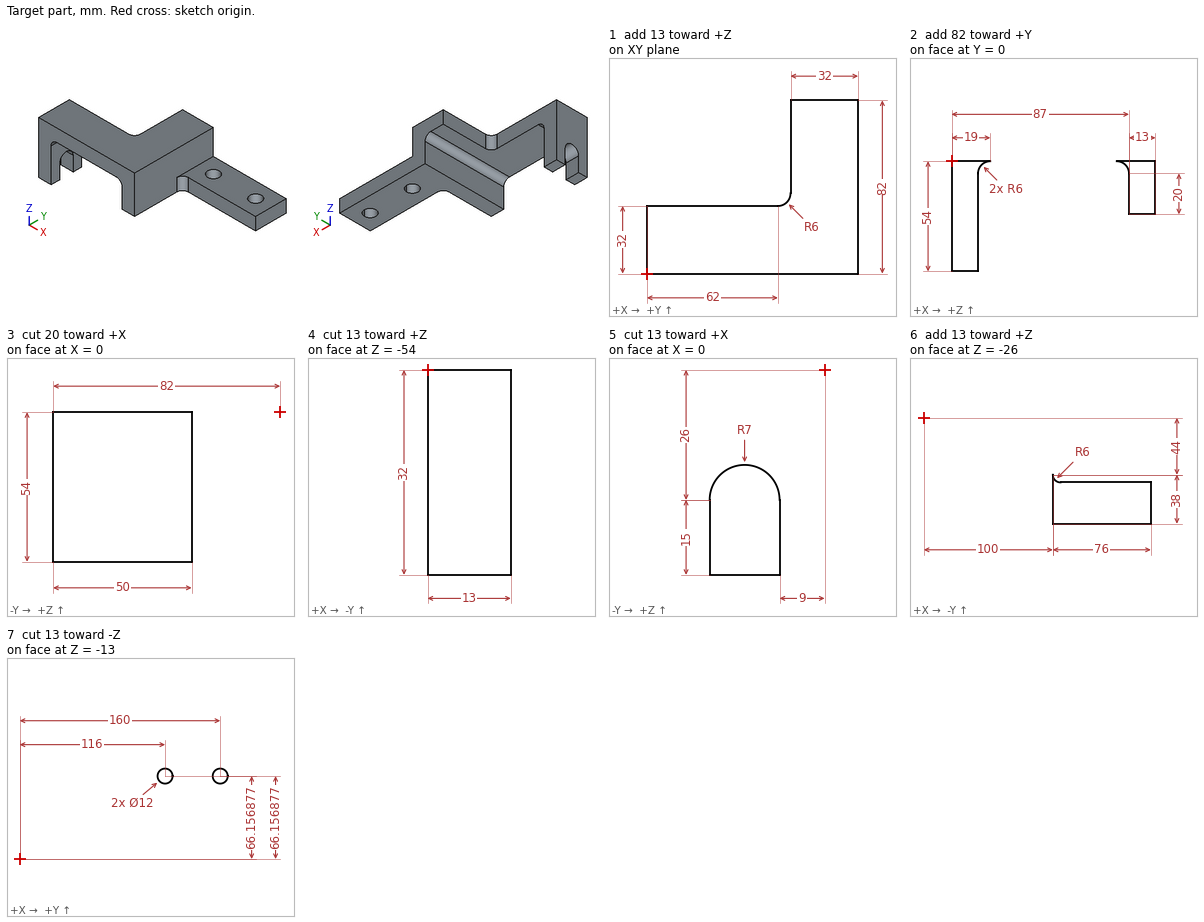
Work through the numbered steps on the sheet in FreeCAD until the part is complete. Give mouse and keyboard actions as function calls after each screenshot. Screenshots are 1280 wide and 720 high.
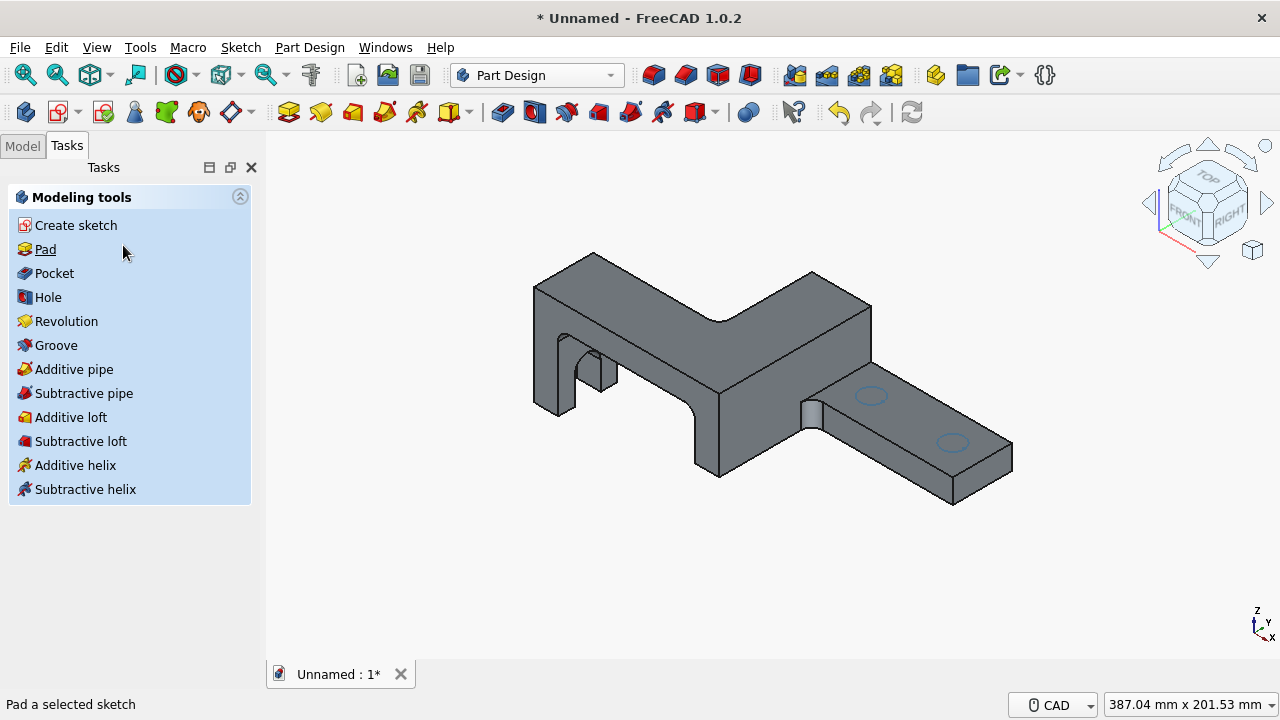
click(504, 112)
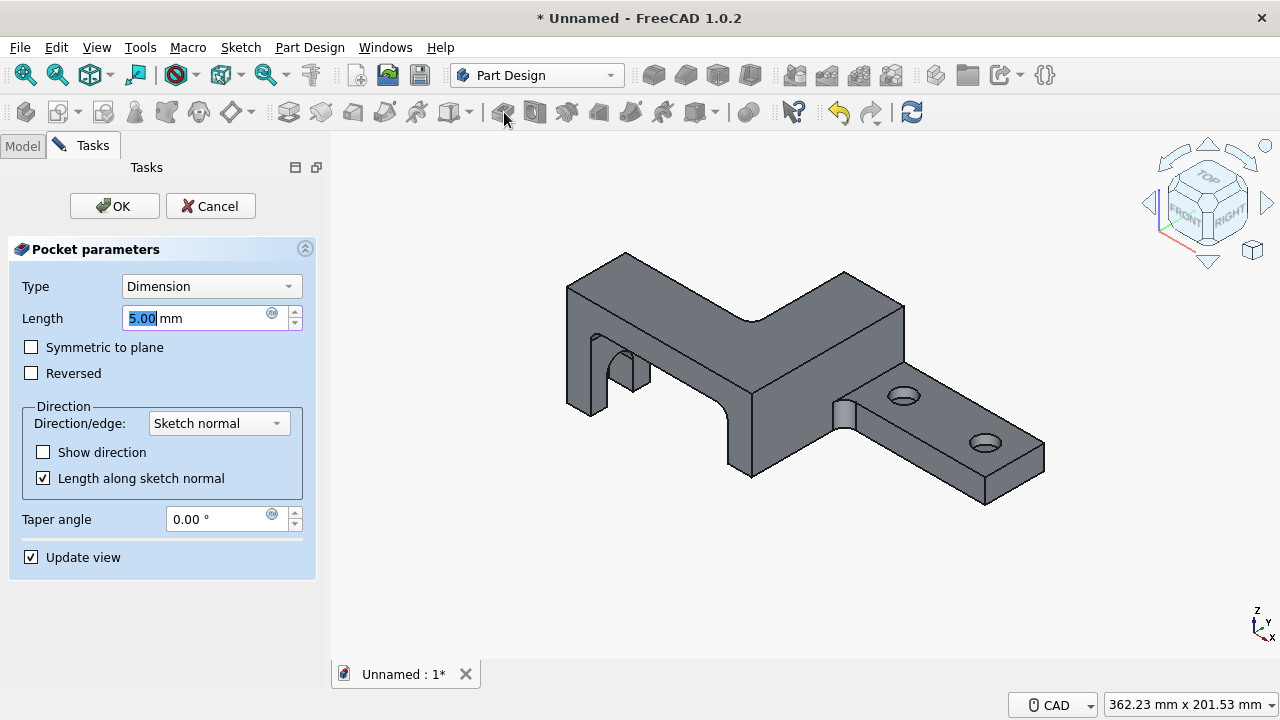
text(13)
key(Tab)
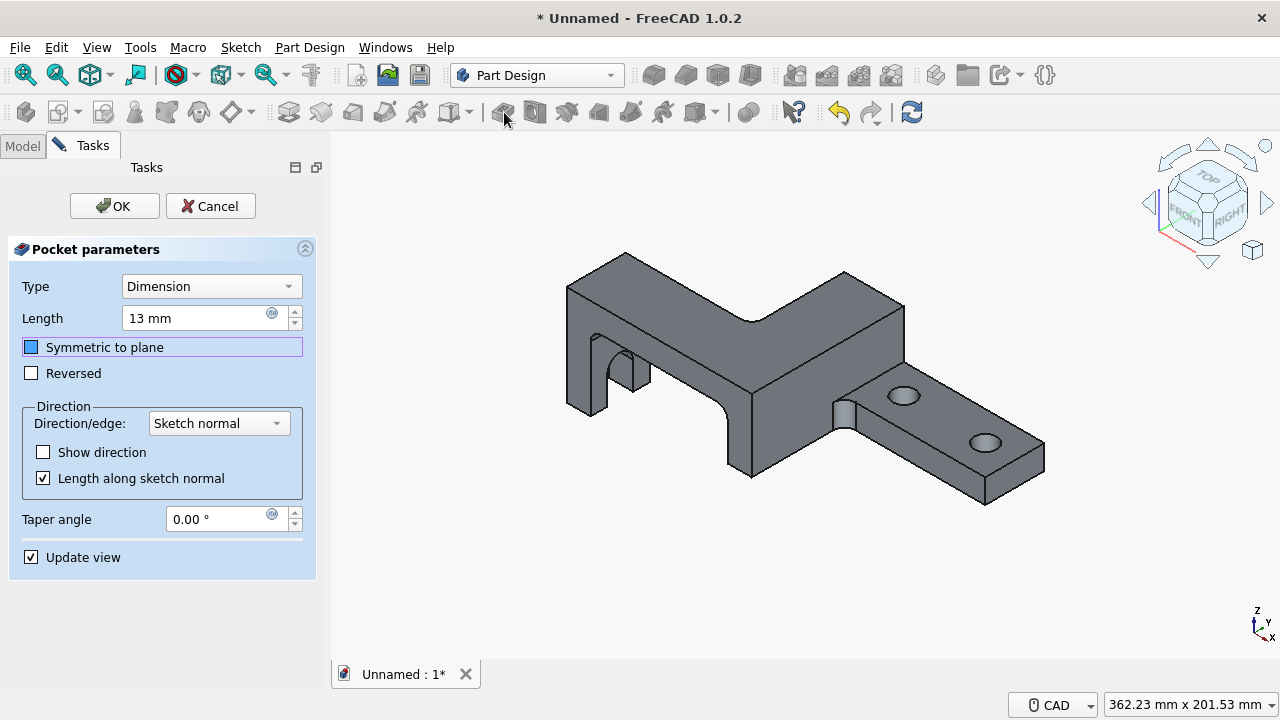
click(115, 206)